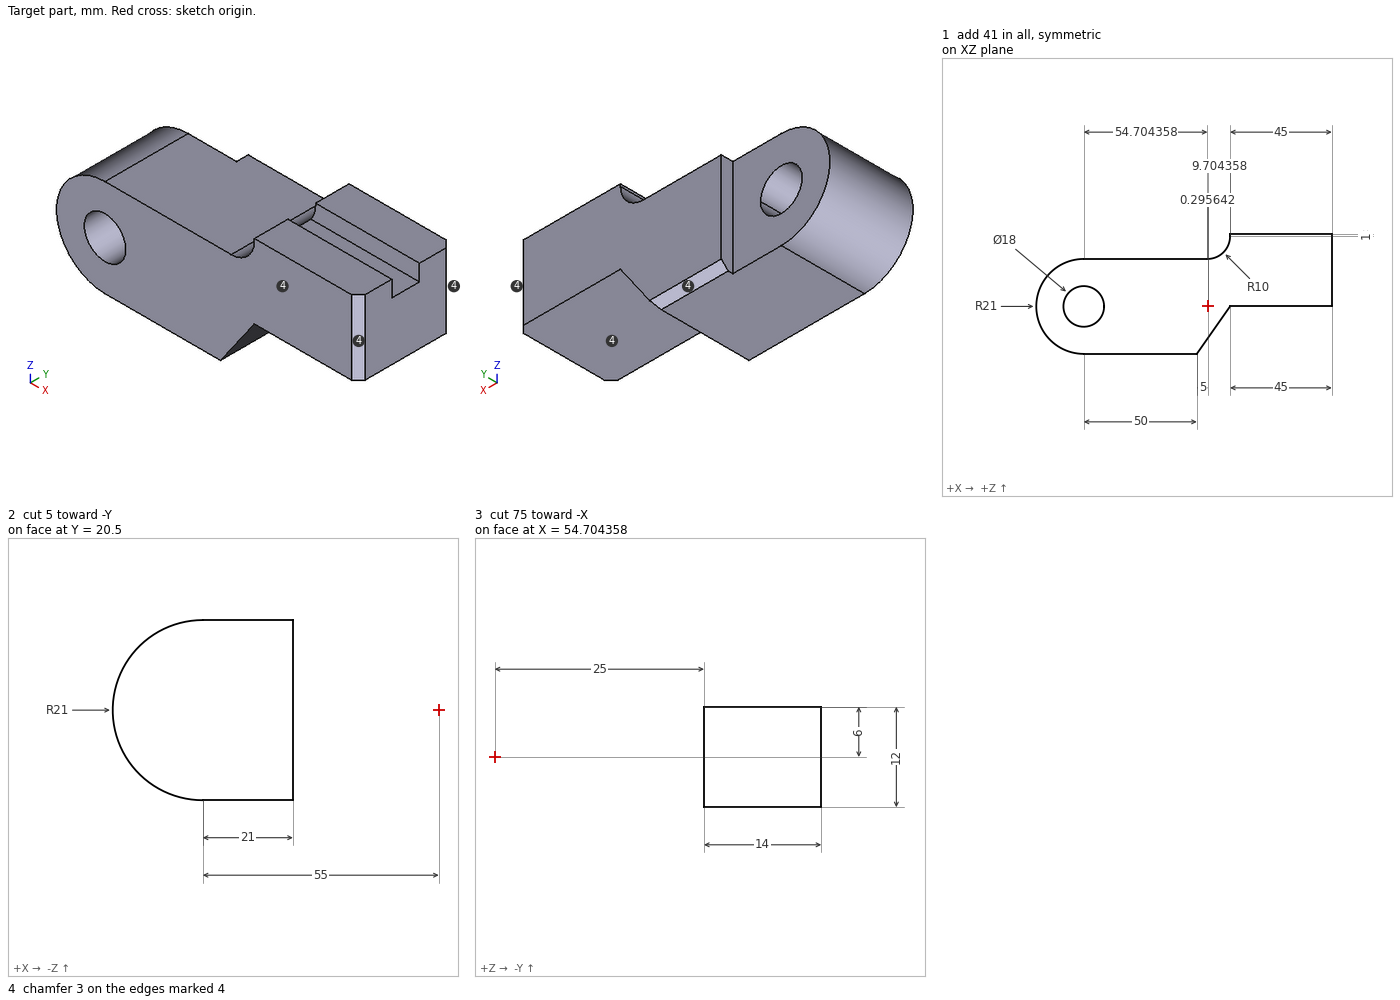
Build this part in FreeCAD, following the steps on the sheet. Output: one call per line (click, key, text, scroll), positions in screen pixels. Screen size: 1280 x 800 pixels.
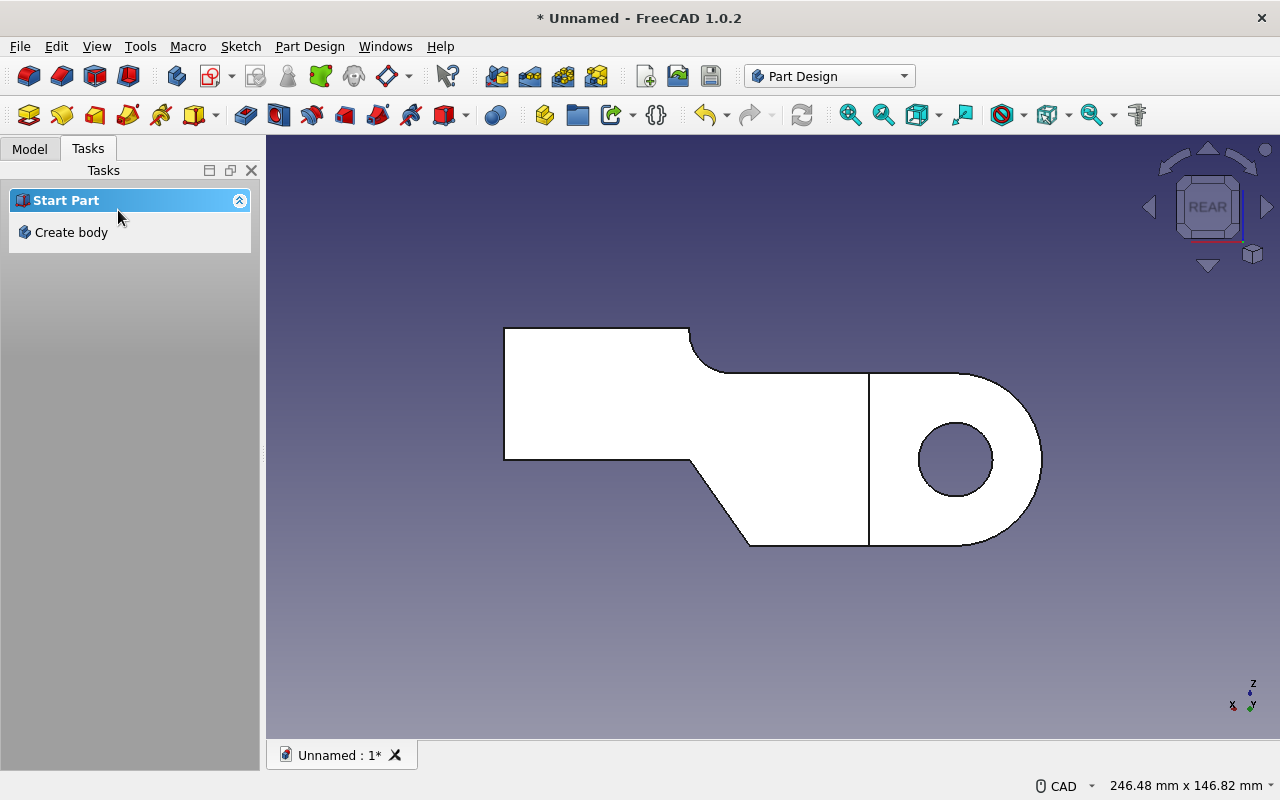
key(0)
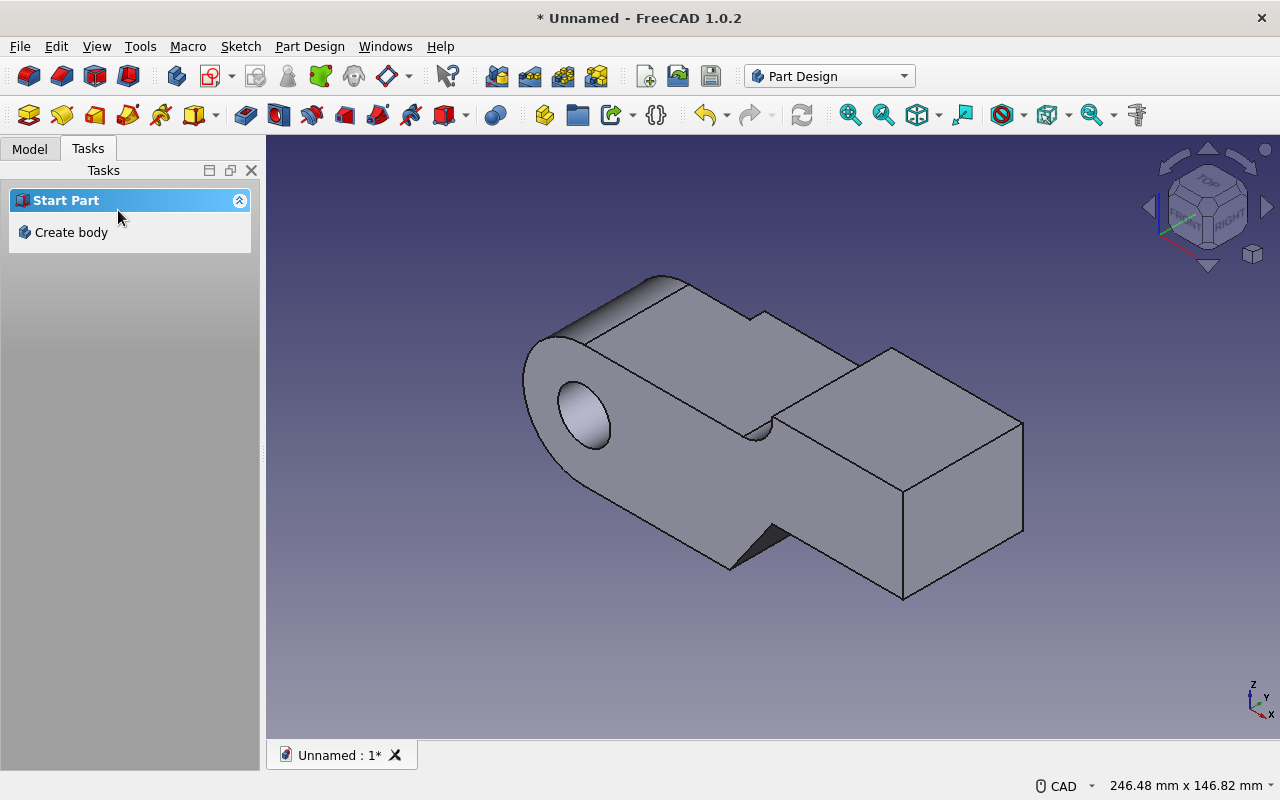
click(963, 510)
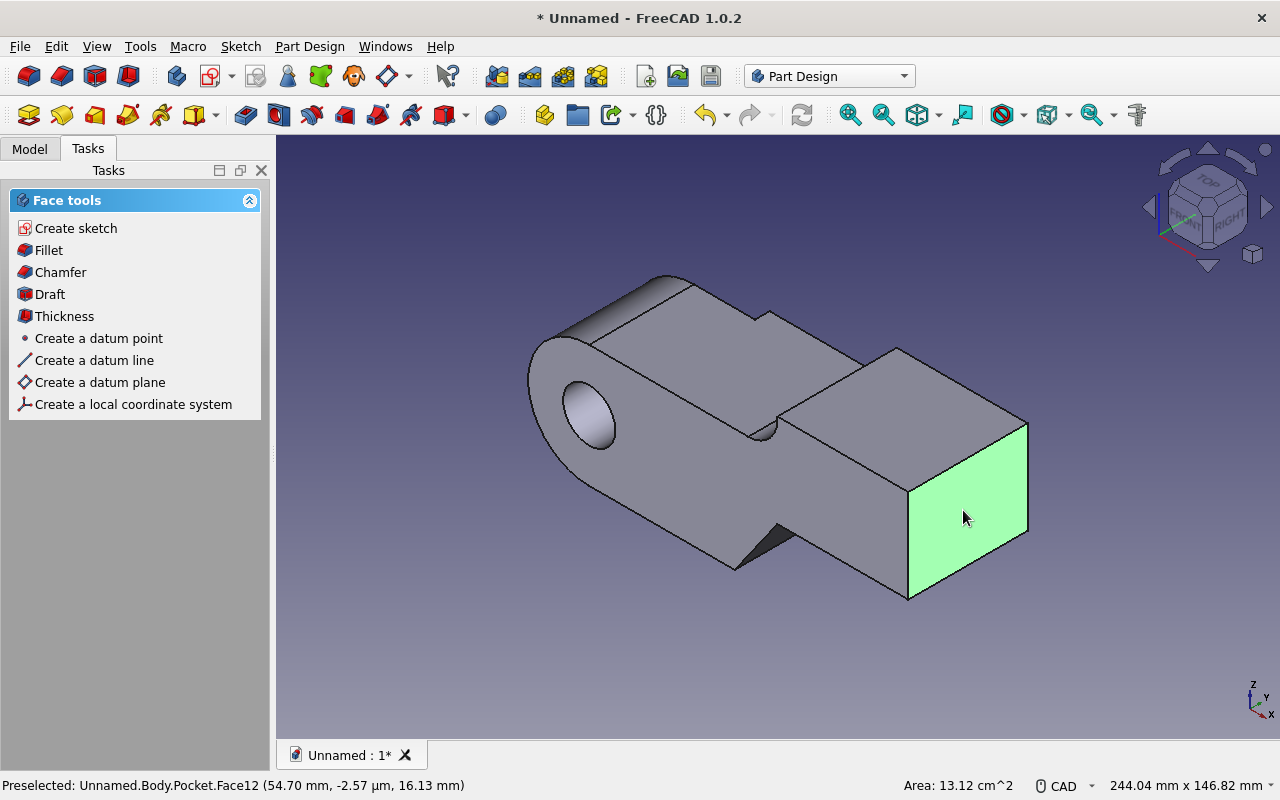
click(210, 76)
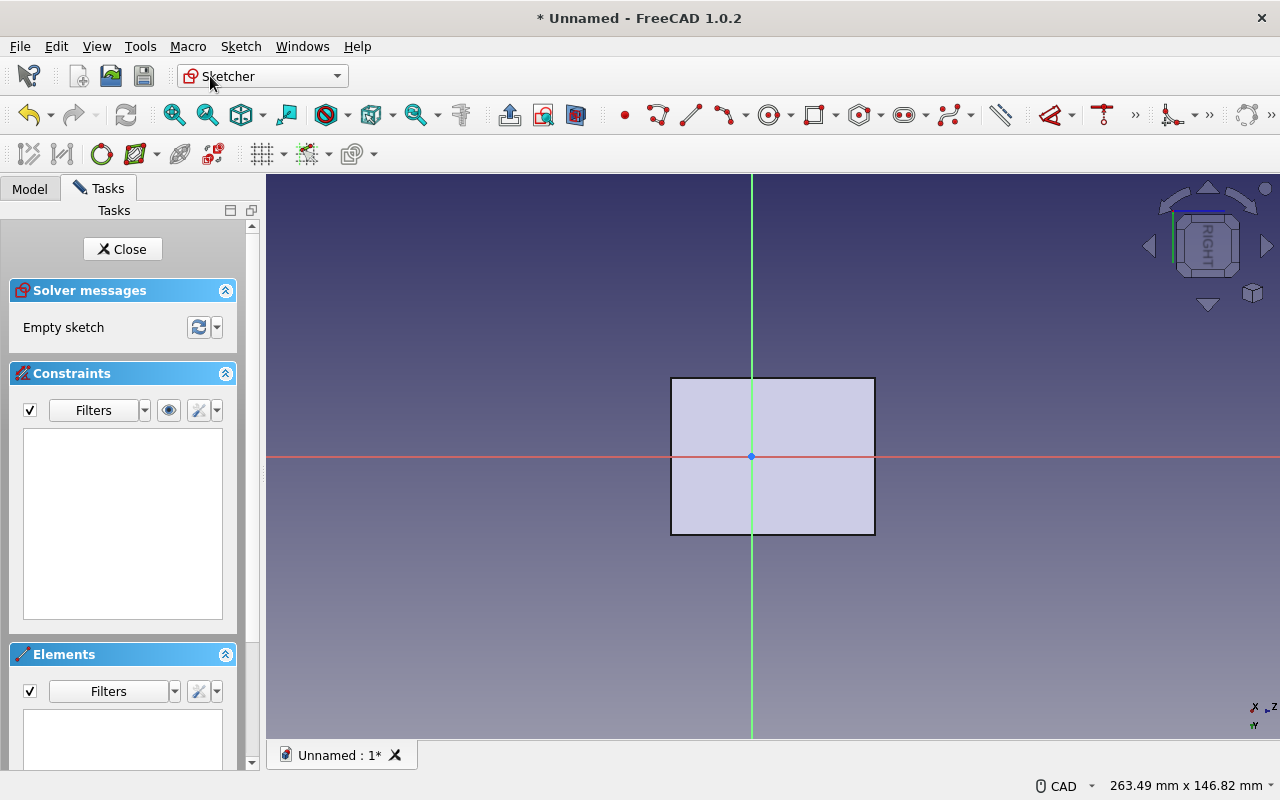
scroll(902, 457, up, 10)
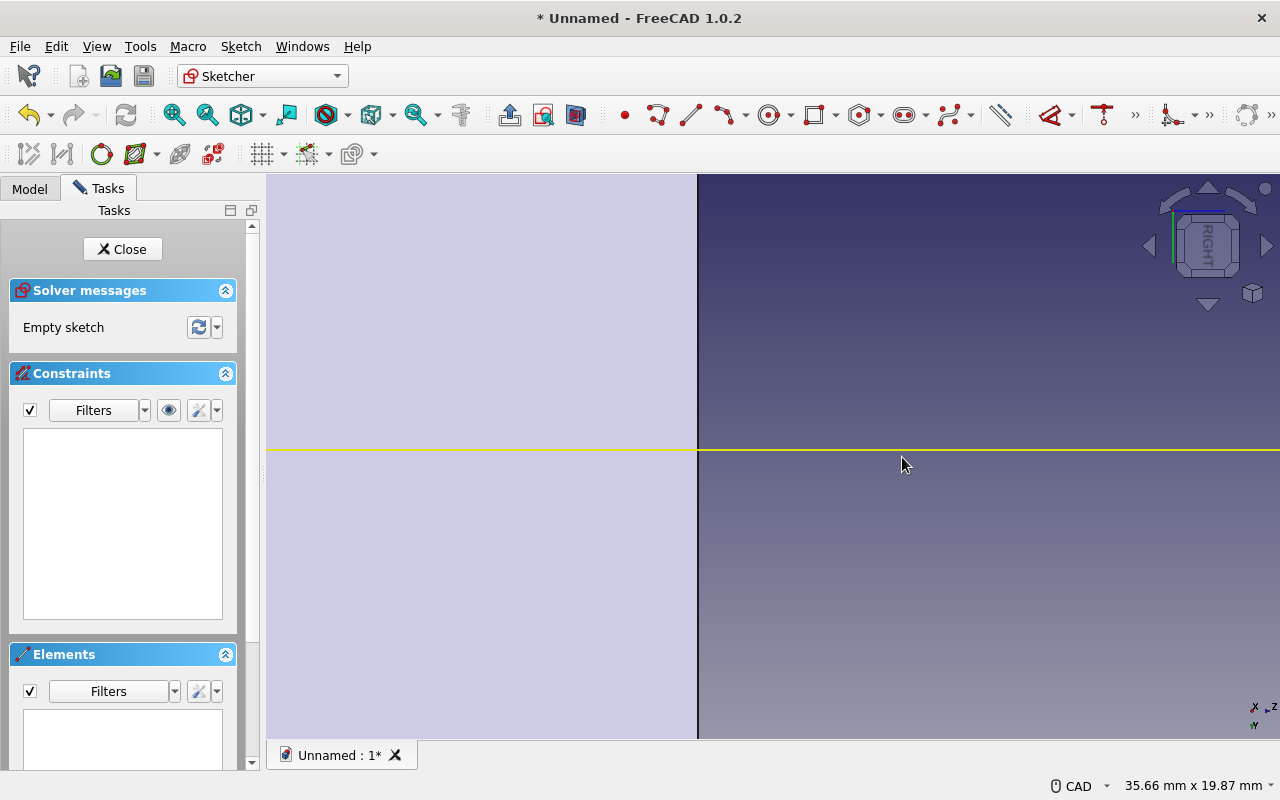
key(g)
key(r)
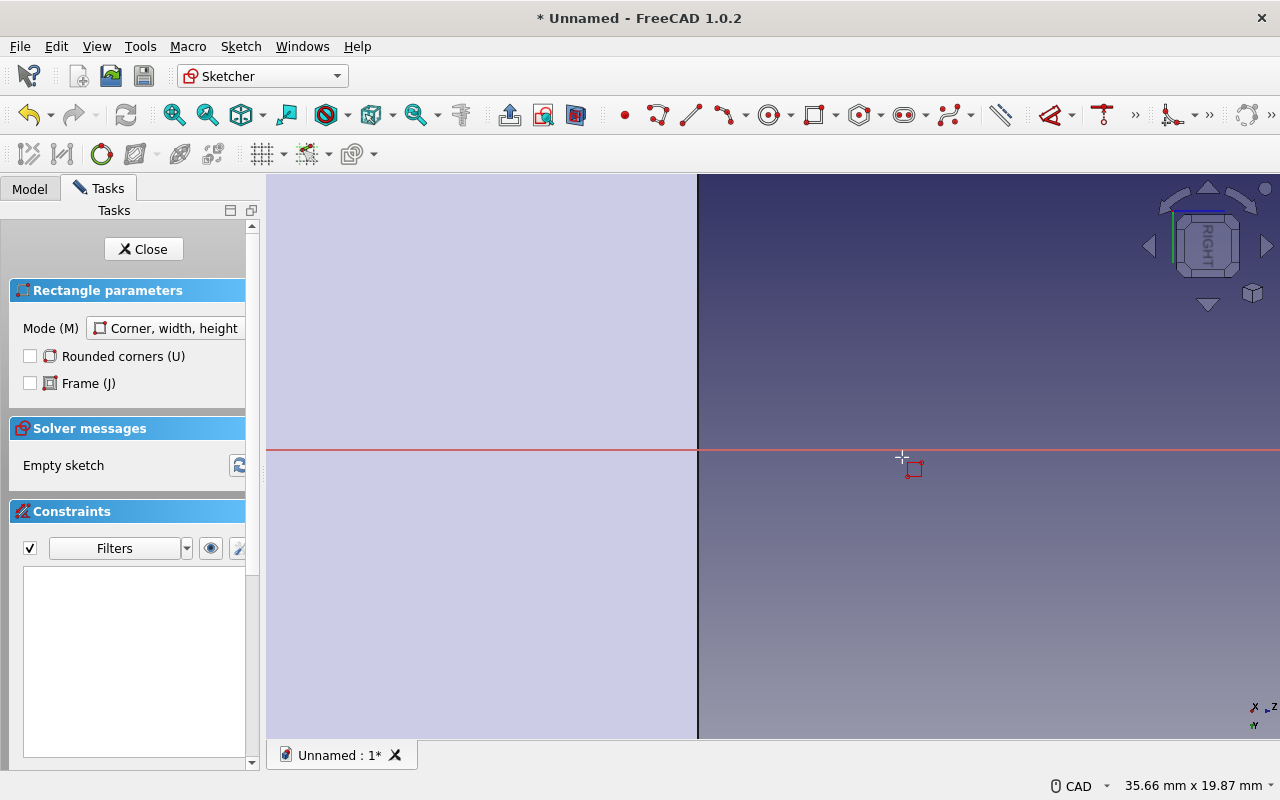
click(499, 279)
click(897, 621)
key(Escape)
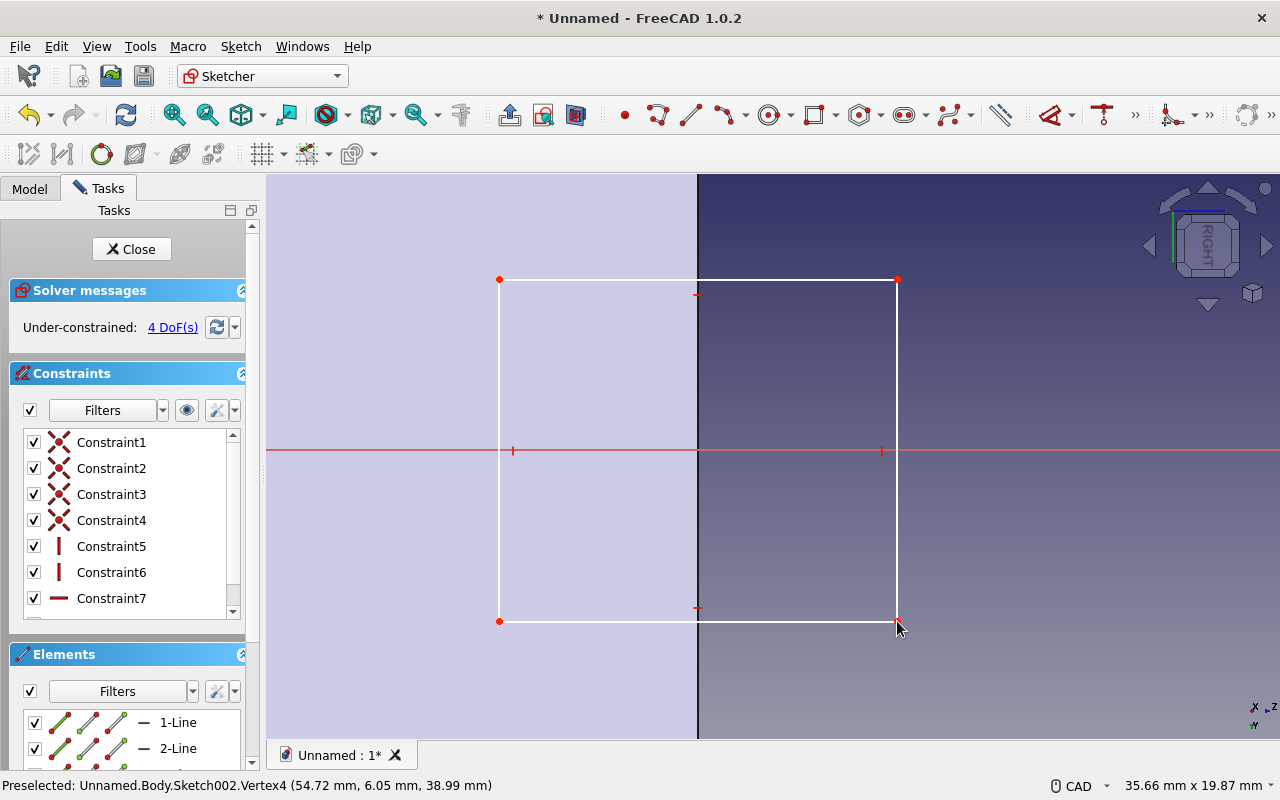
click(1050, 116)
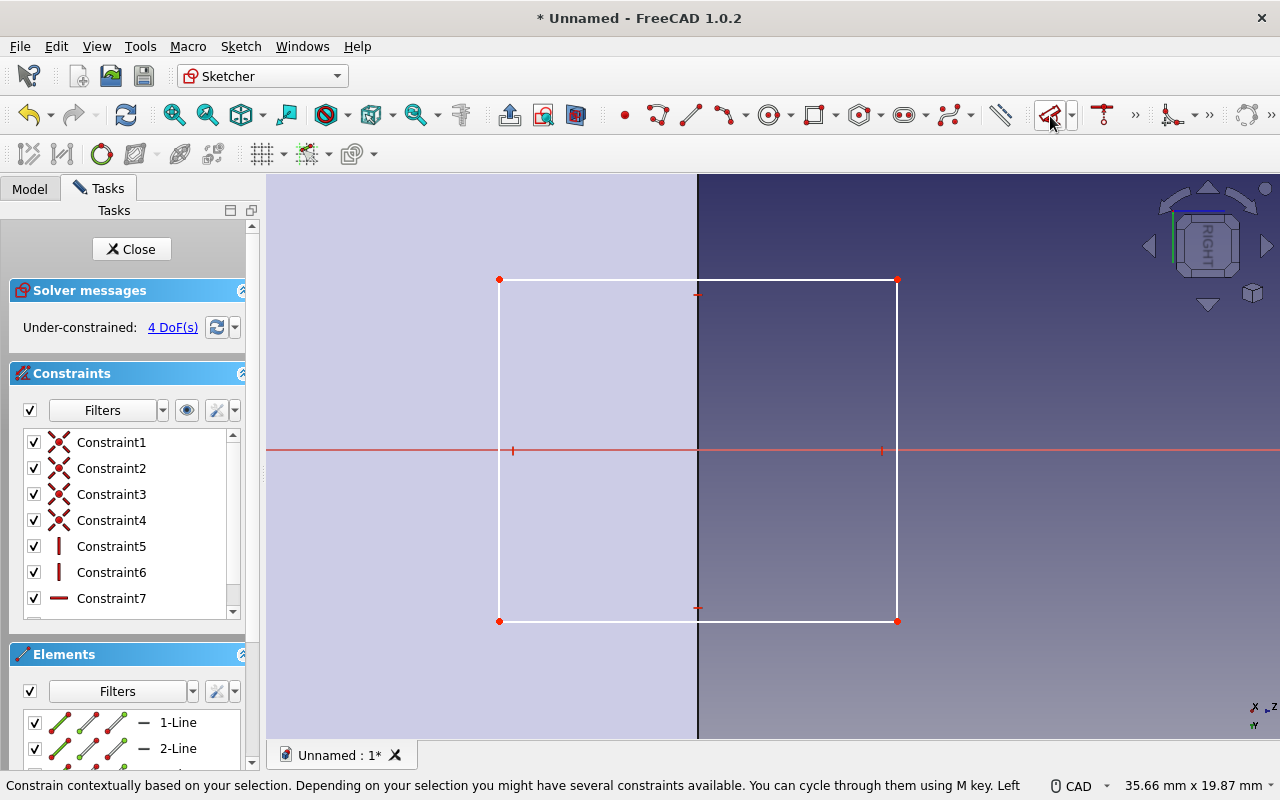
click(499, 383)
click(465, 372)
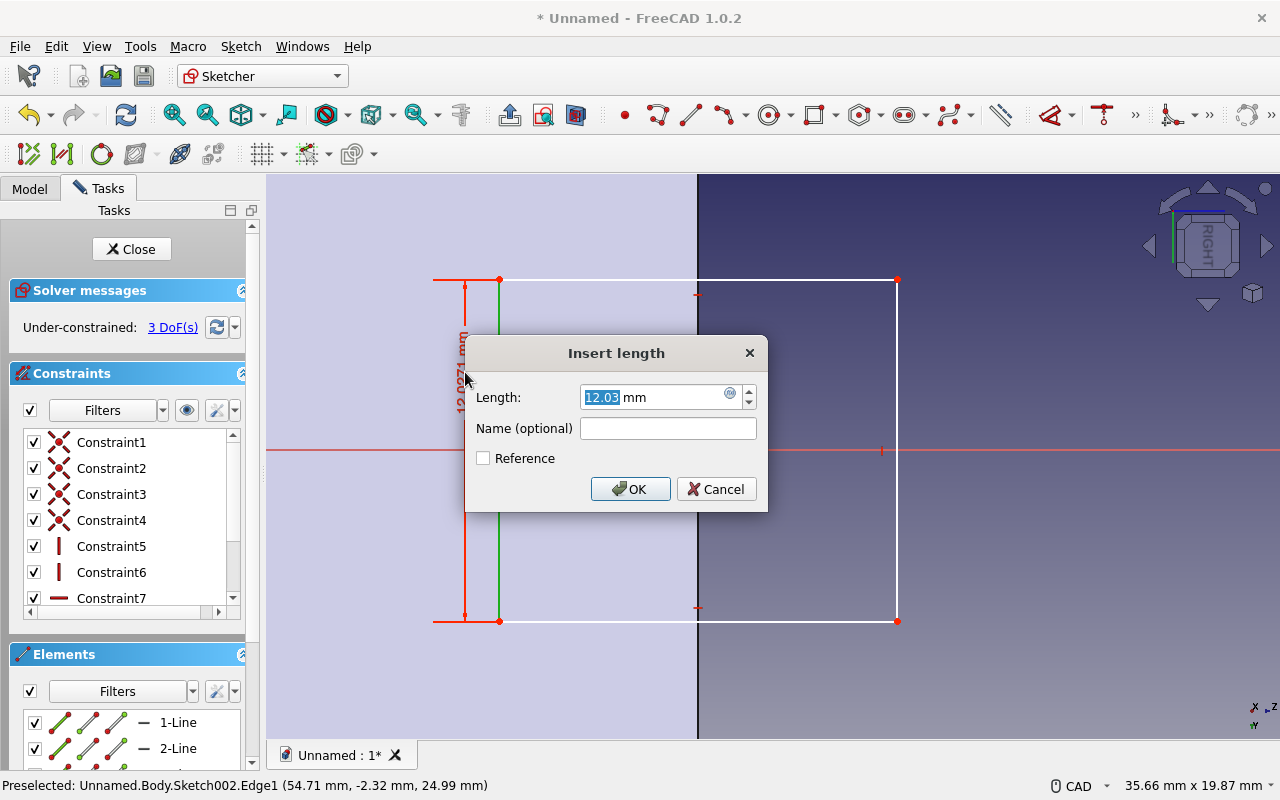
text(12)
key(Return)